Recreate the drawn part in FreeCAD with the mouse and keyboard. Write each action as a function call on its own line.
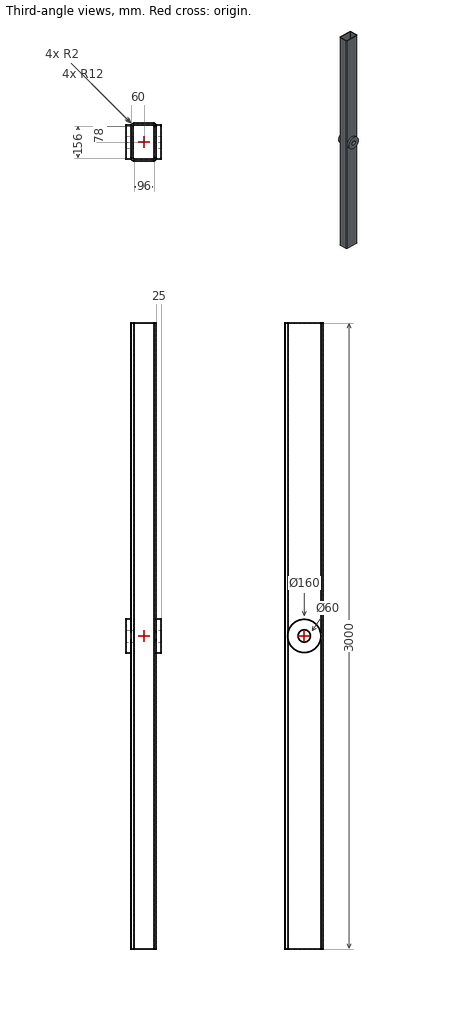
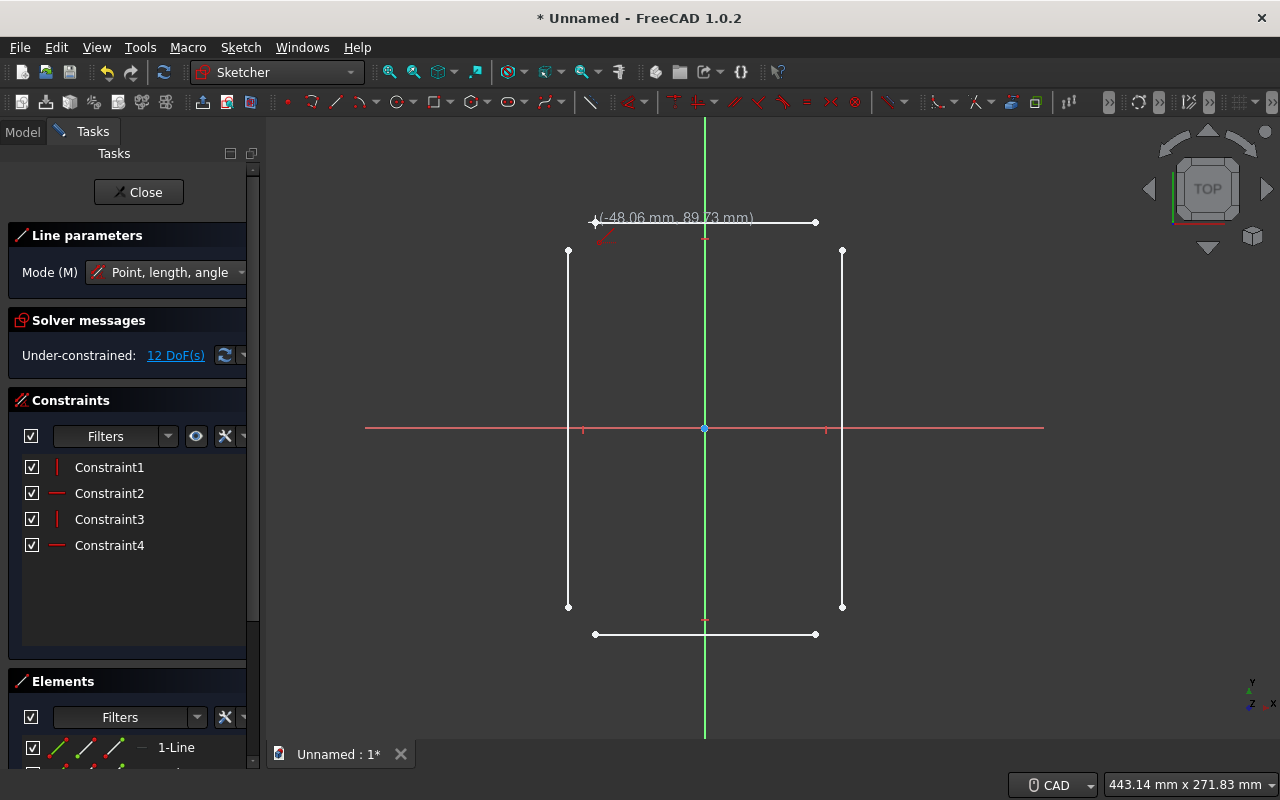
key(g)
key(3)
key(a)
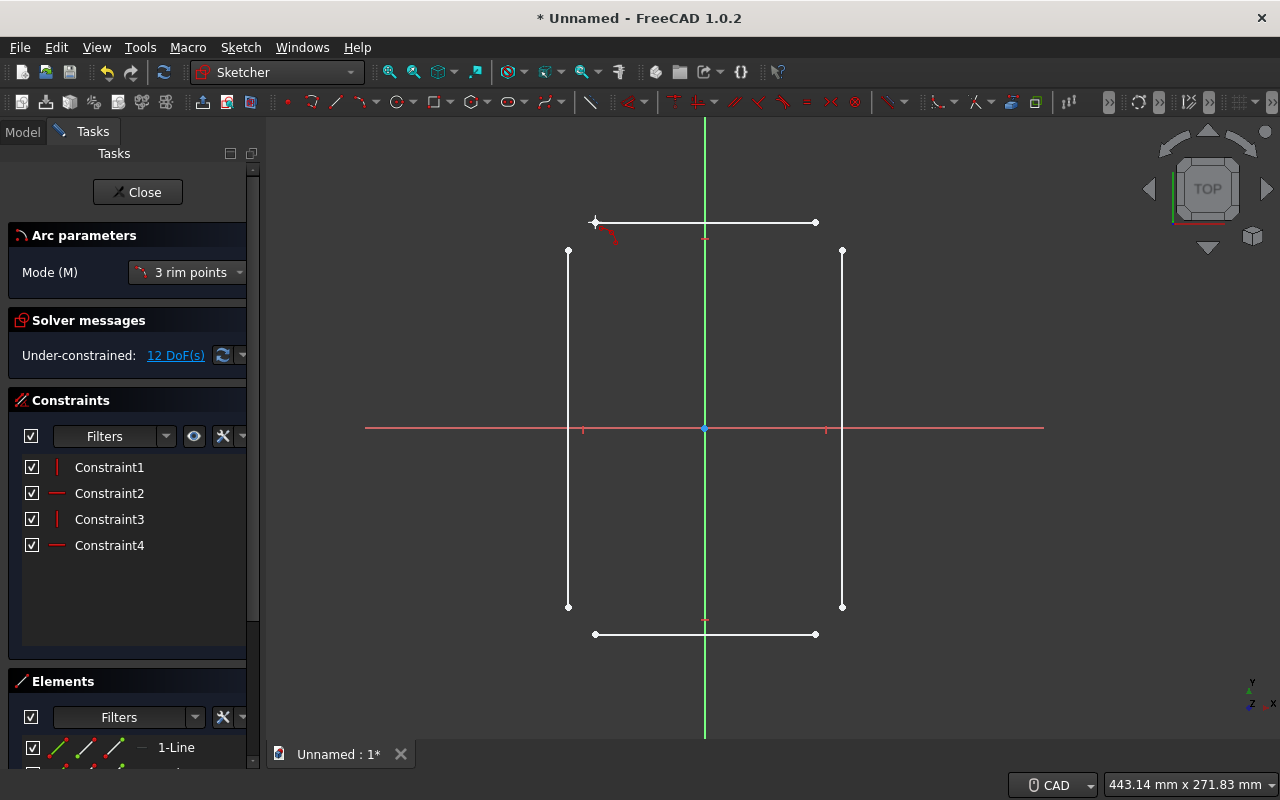
click(568, 608)
click(595, 635)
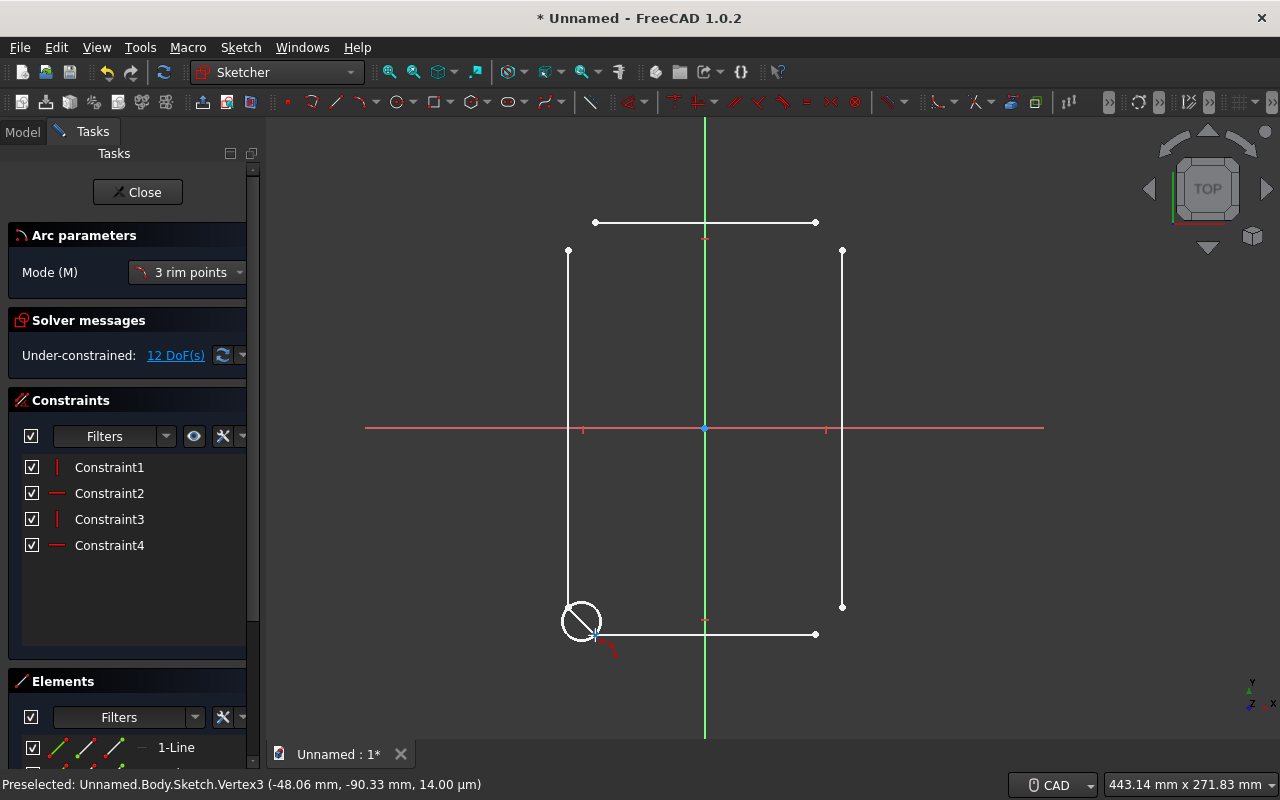
scroll(576, 626, up, 4)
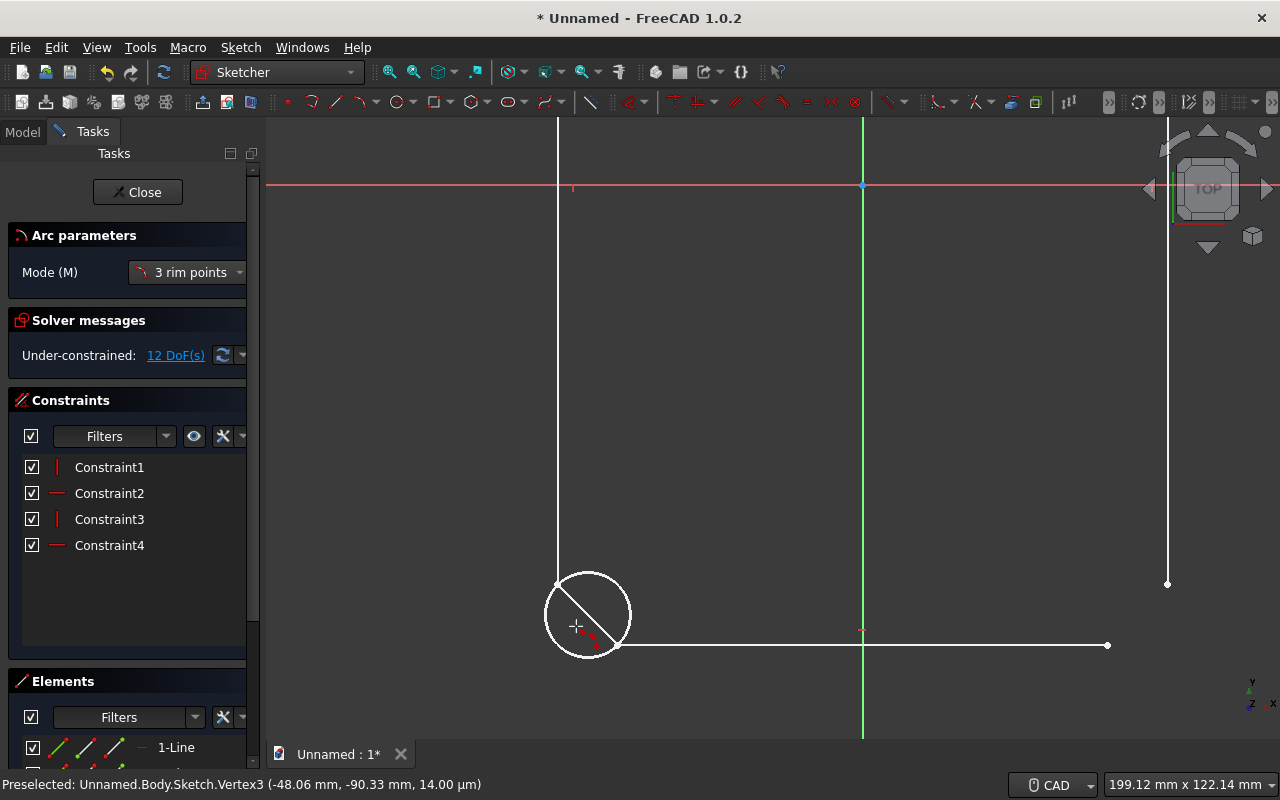
click(575, 625)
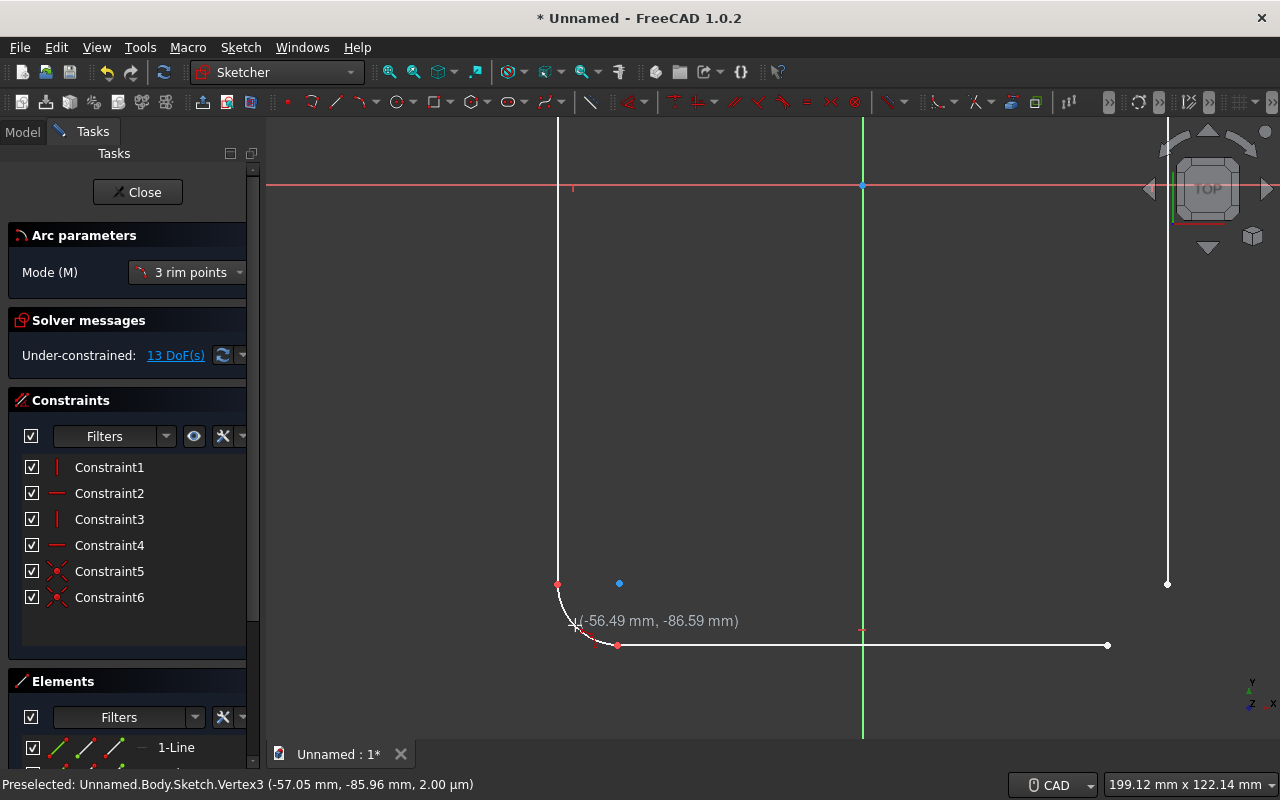
click(1108, 645)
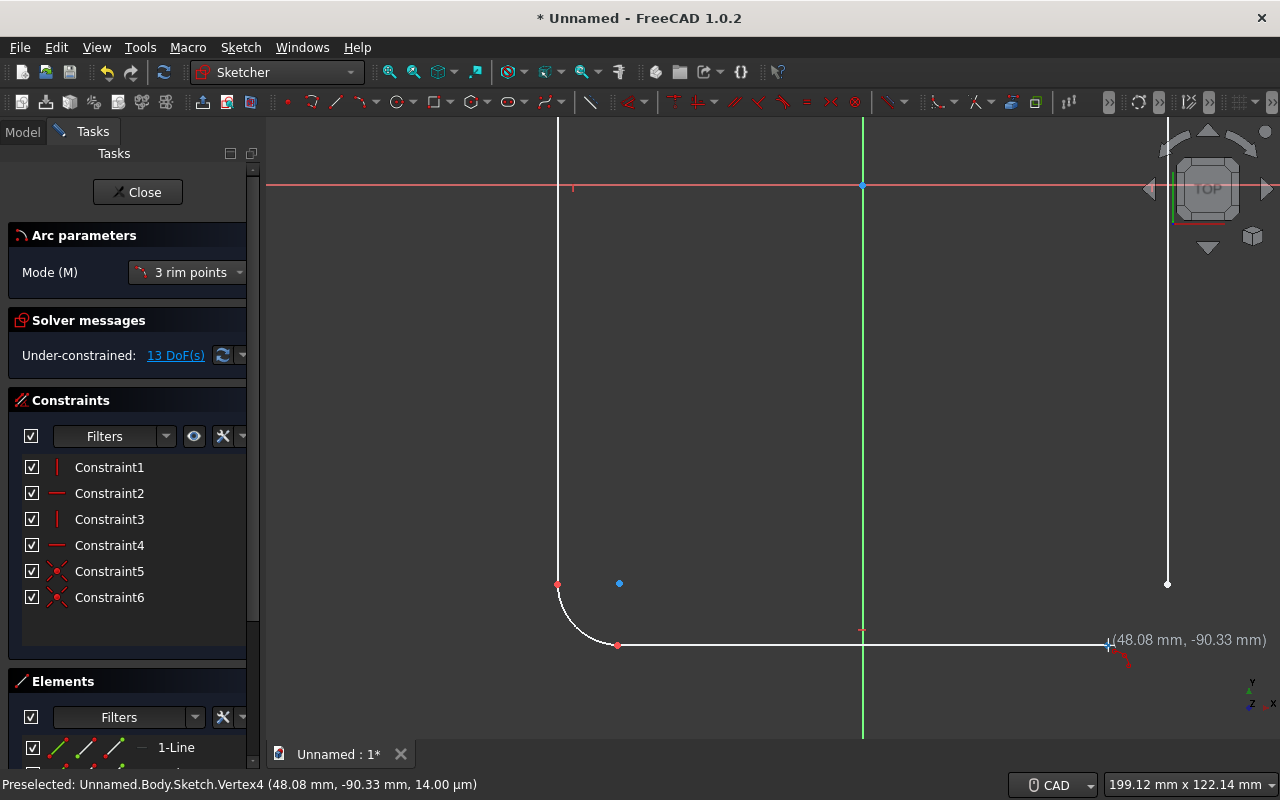
scroll(575, 626, down, 4)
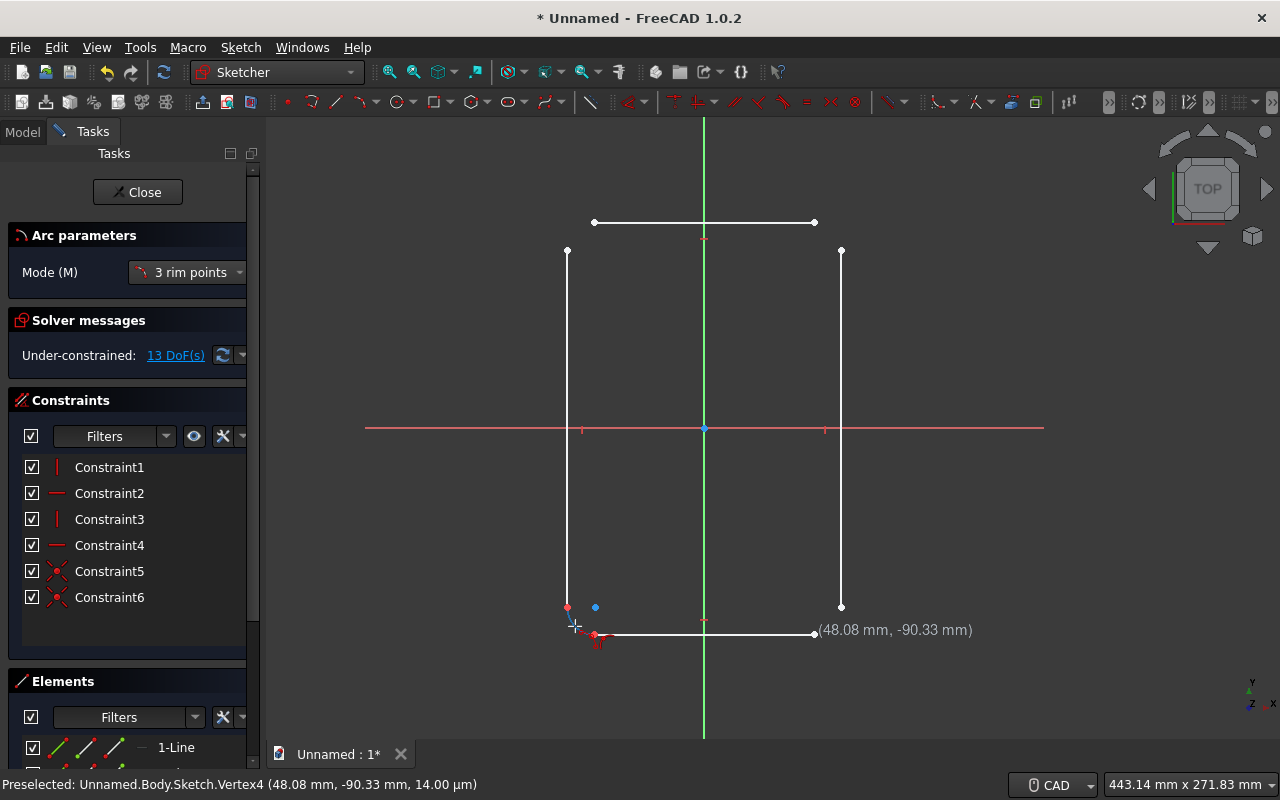
click(841, 608)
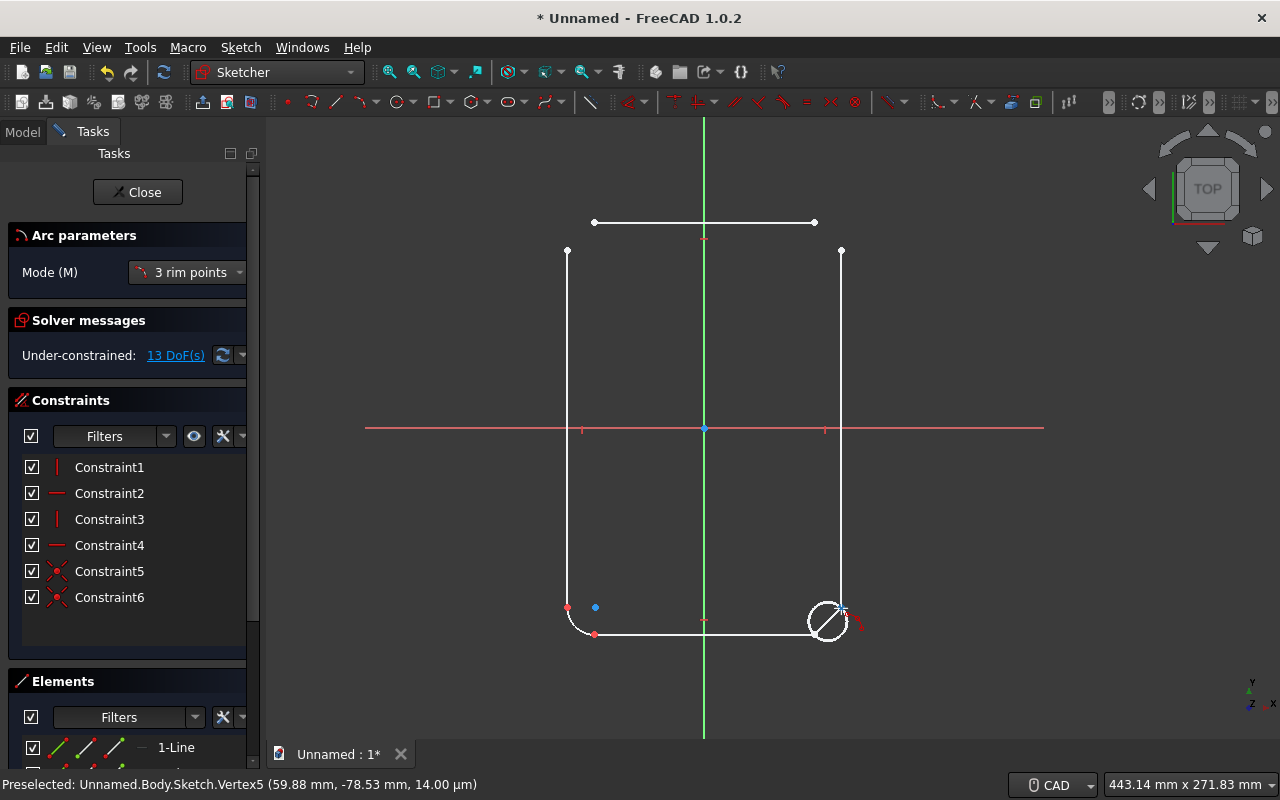
scroll(834, 626, up, 4)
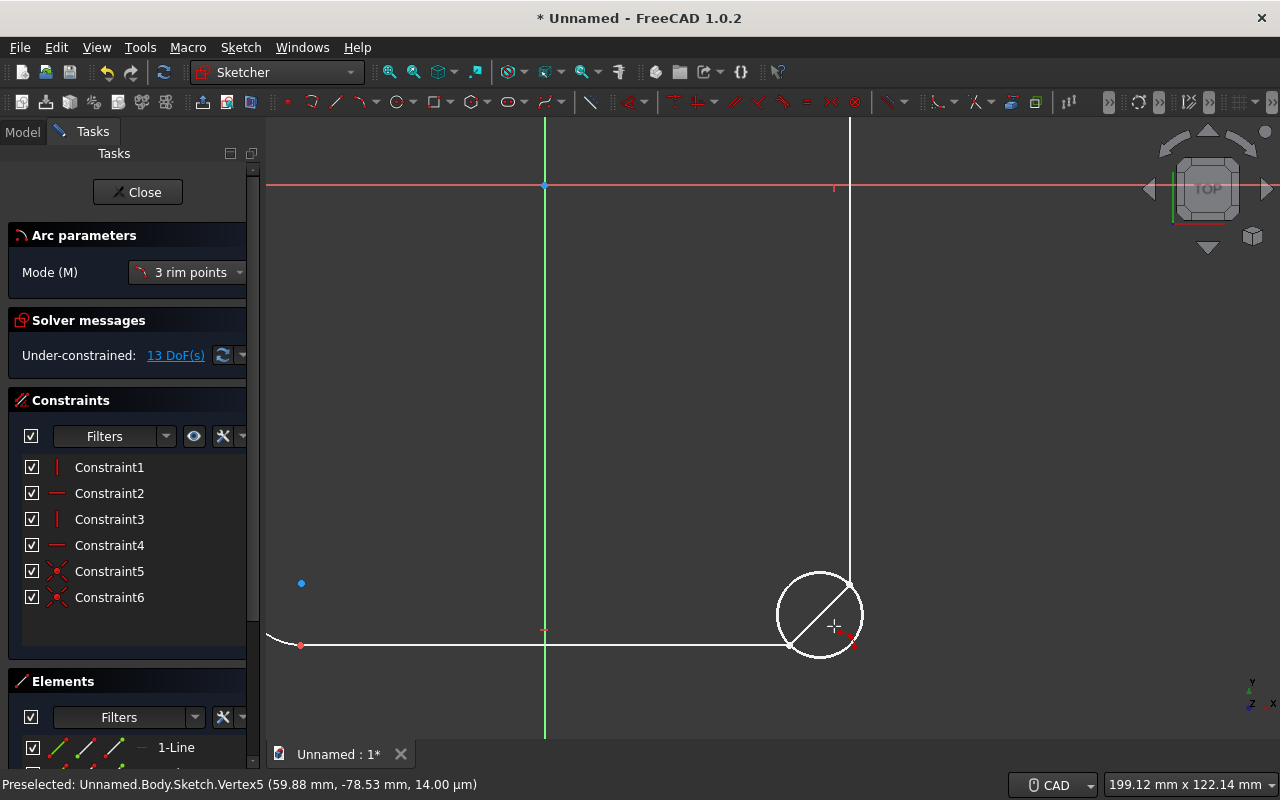
click(833, 625)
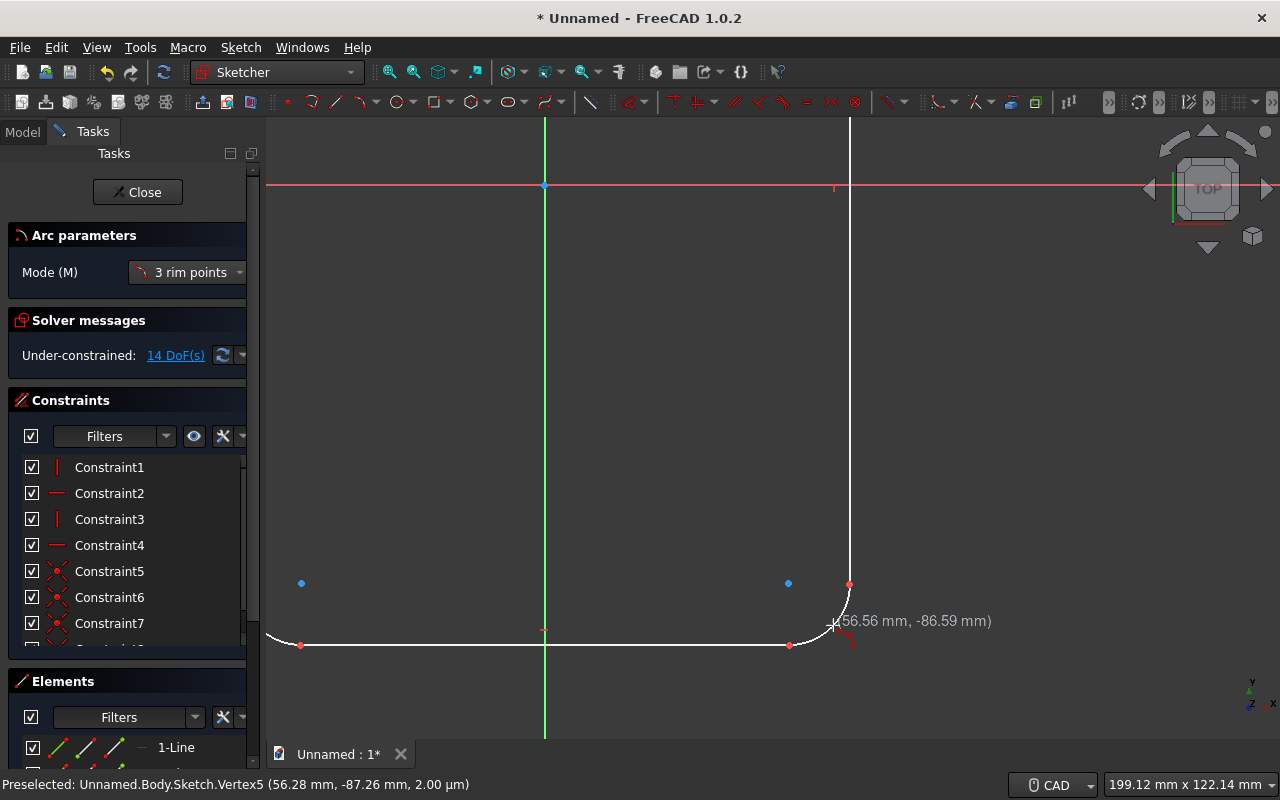
scroll(835, 626, down, 4)